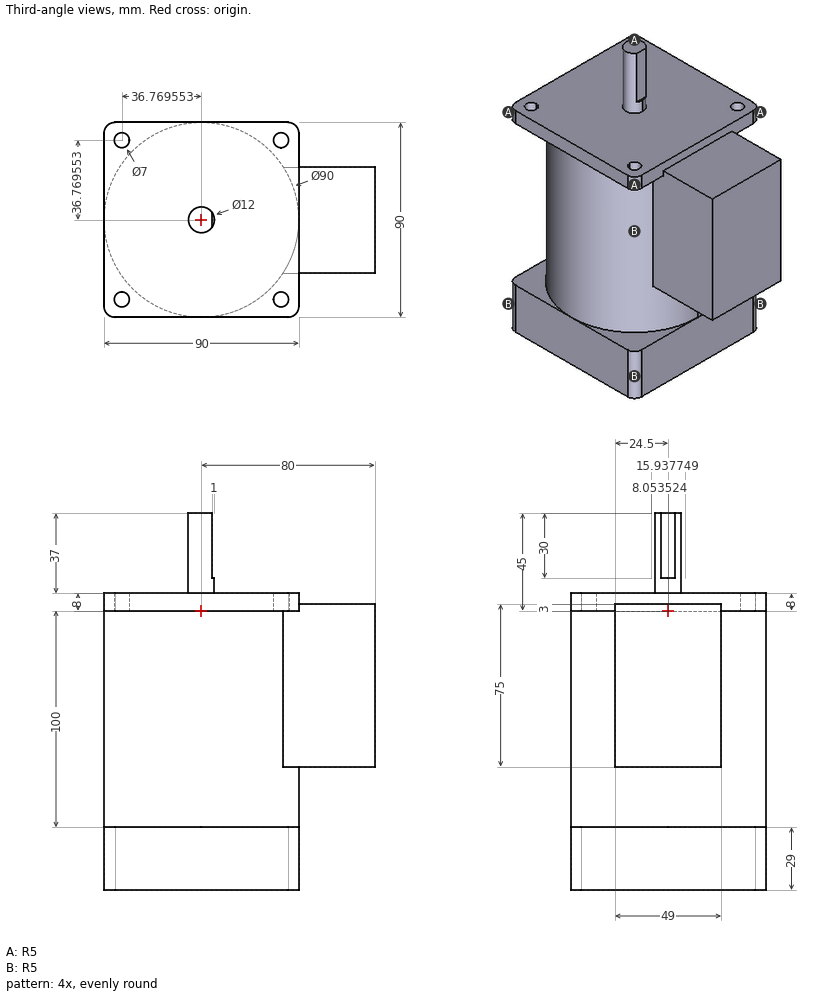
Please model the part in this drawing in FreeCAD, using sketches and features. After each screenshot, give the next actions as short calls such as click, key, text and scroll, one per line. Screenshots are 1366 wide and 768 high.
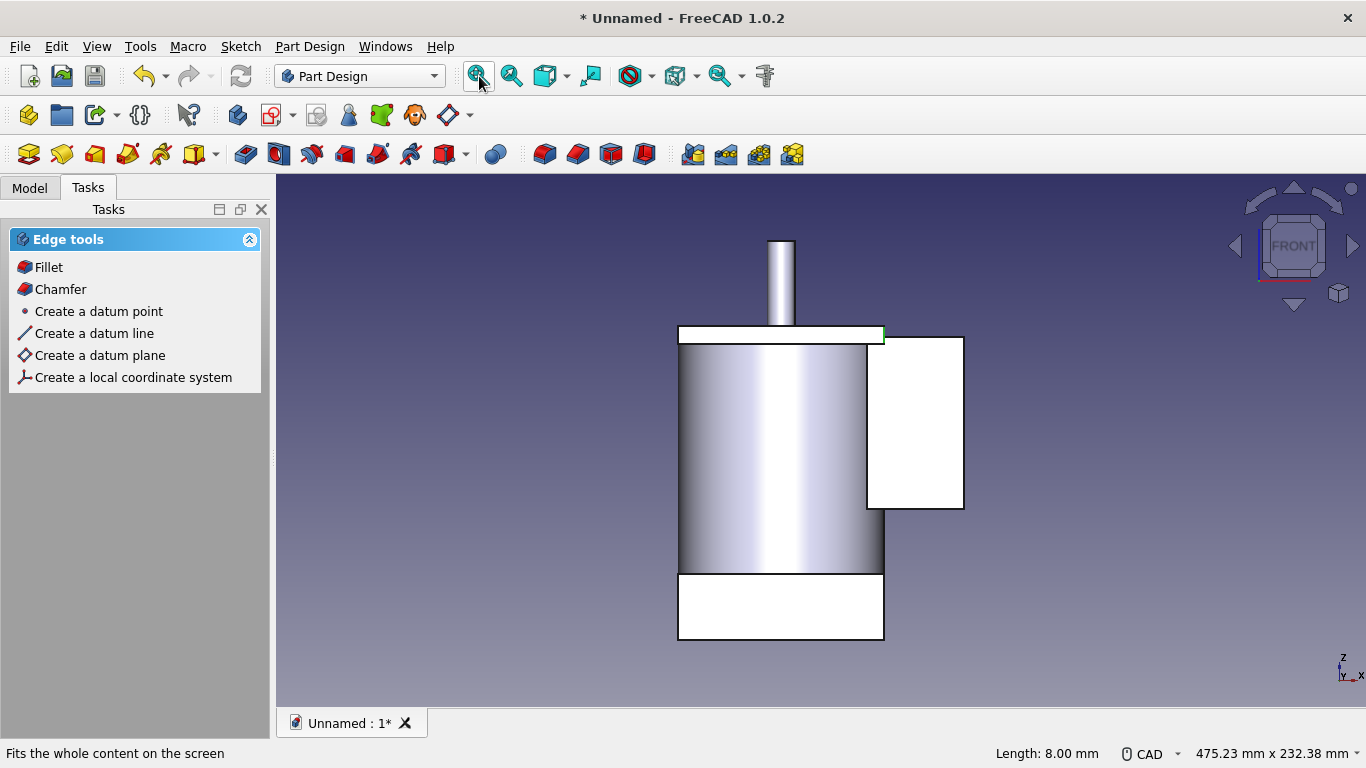
click(678, 334, ctrl)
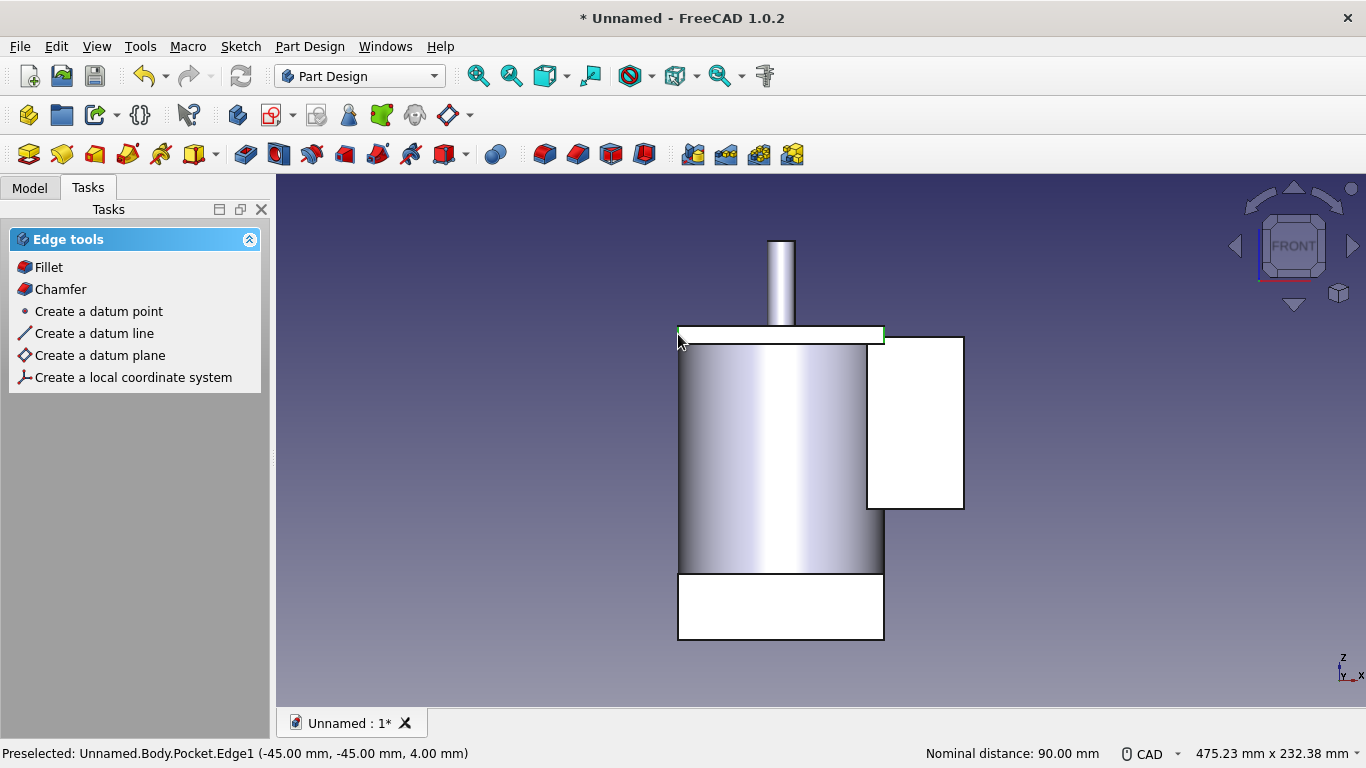
scroll(678, 334, up, 4)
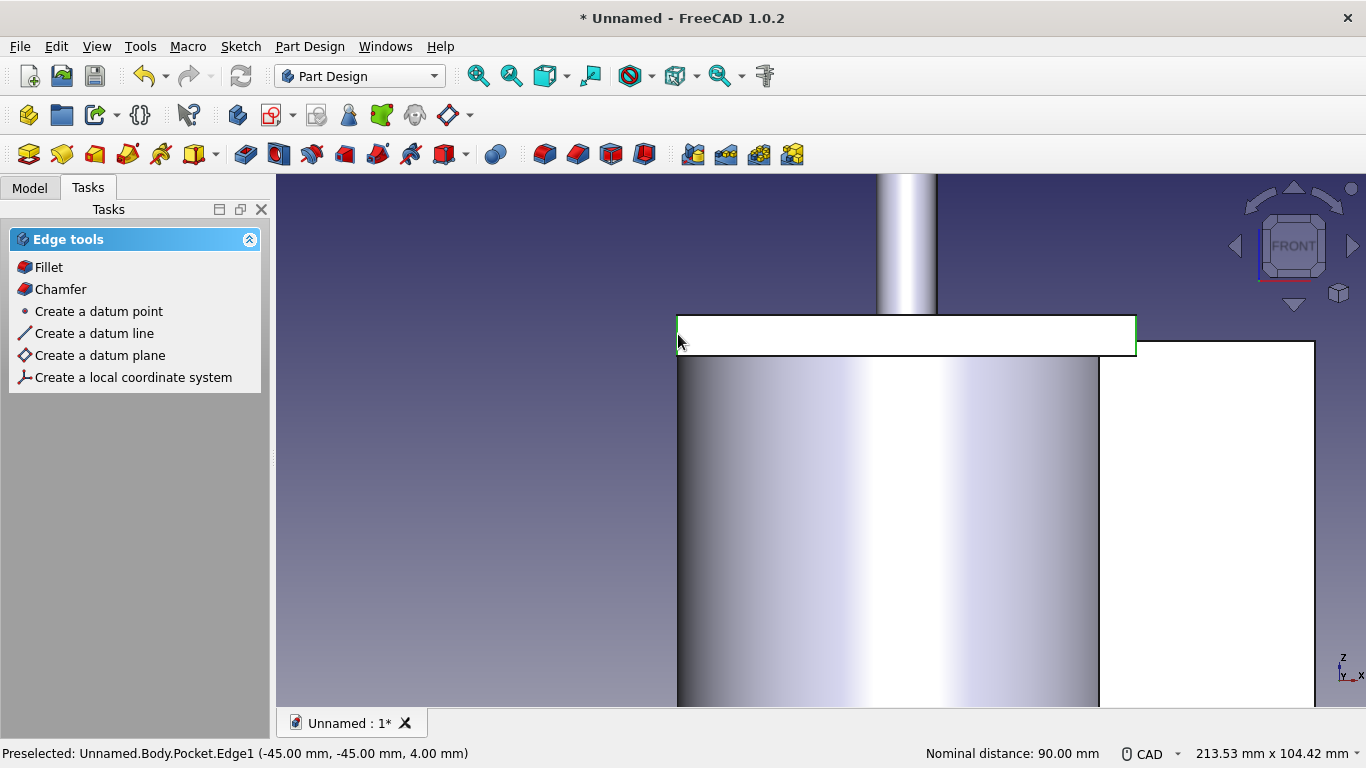
key(v)
key(f)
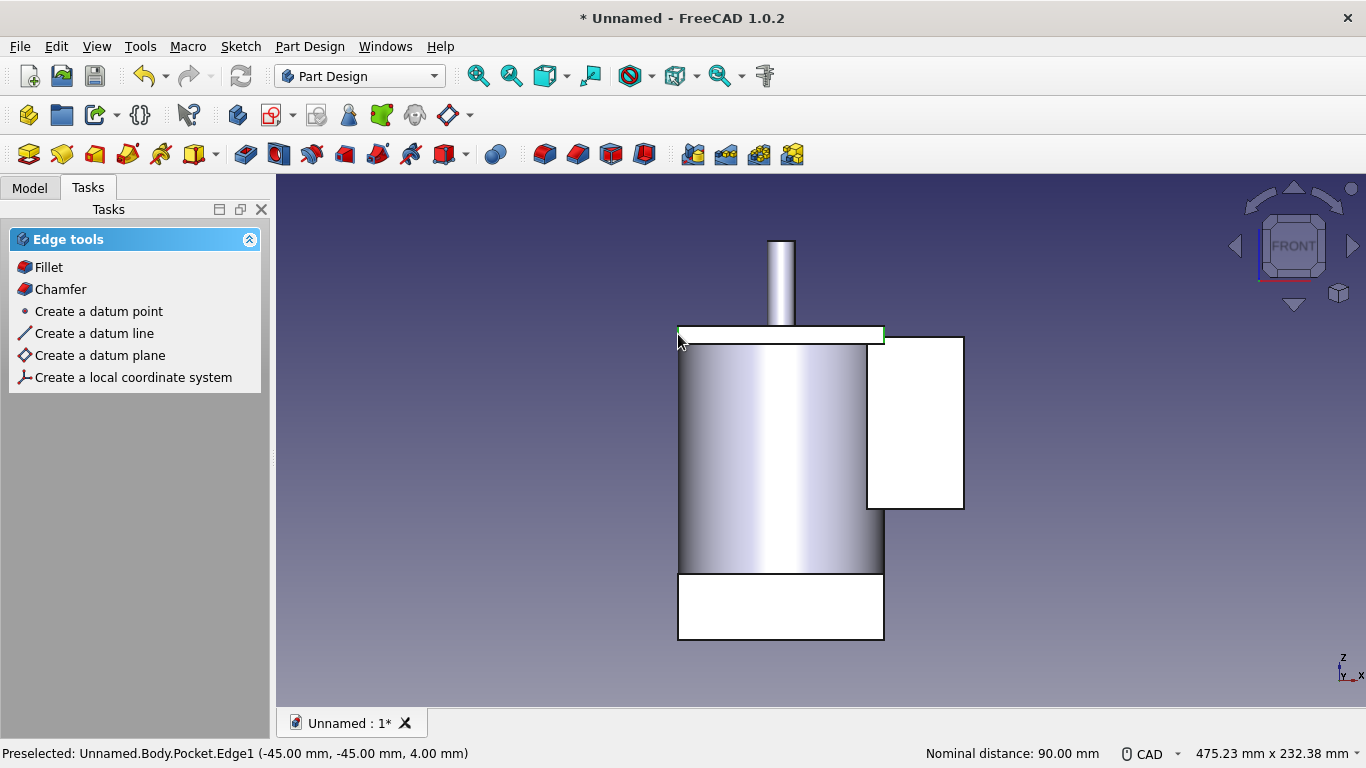
key(3)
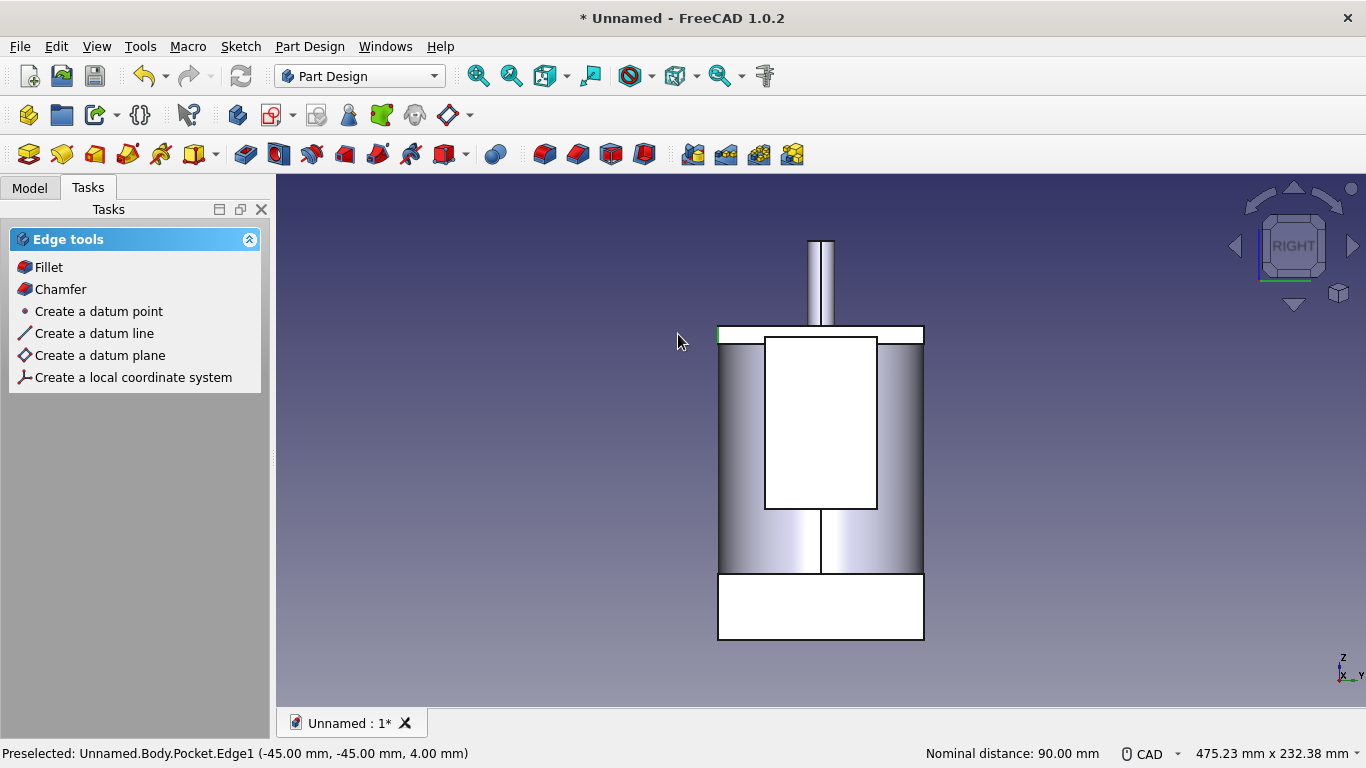
click(924, 334, ctrl)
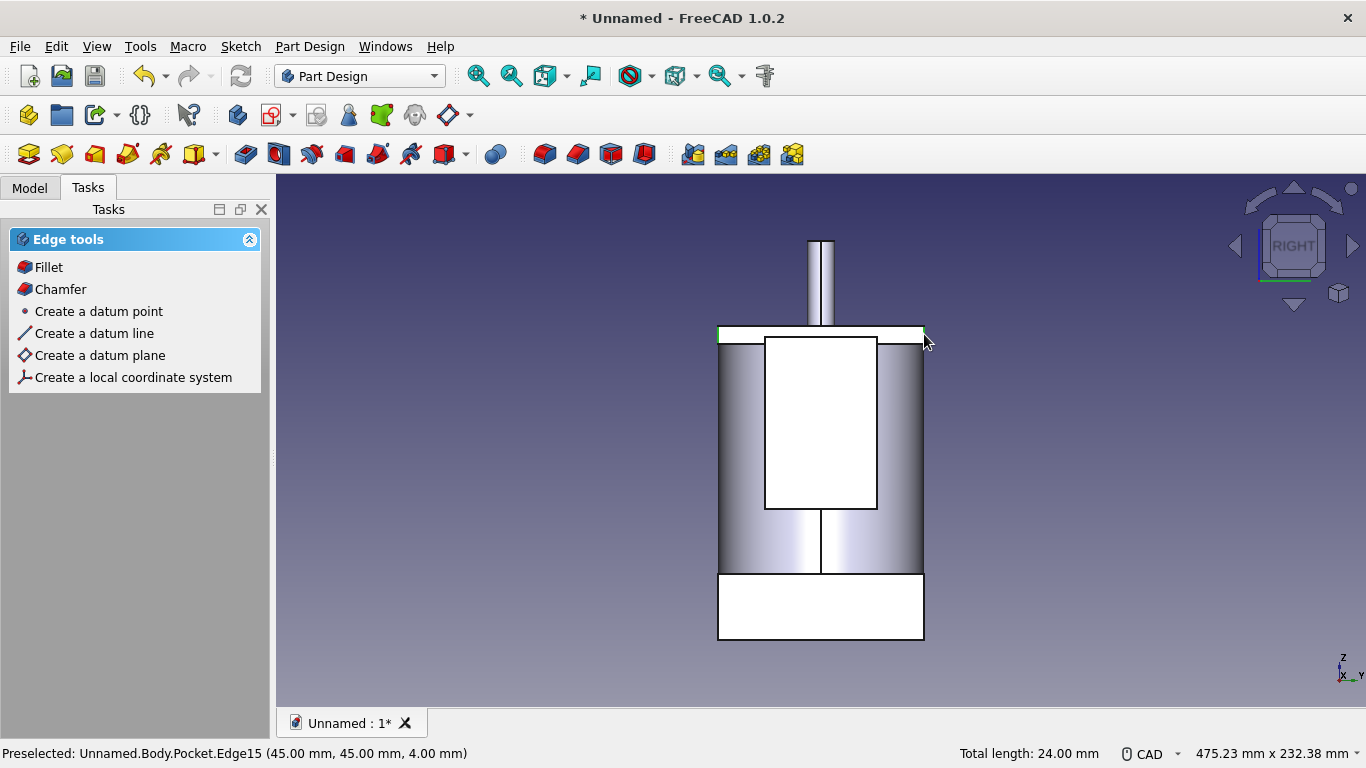
scroll(924, 334, up, 4)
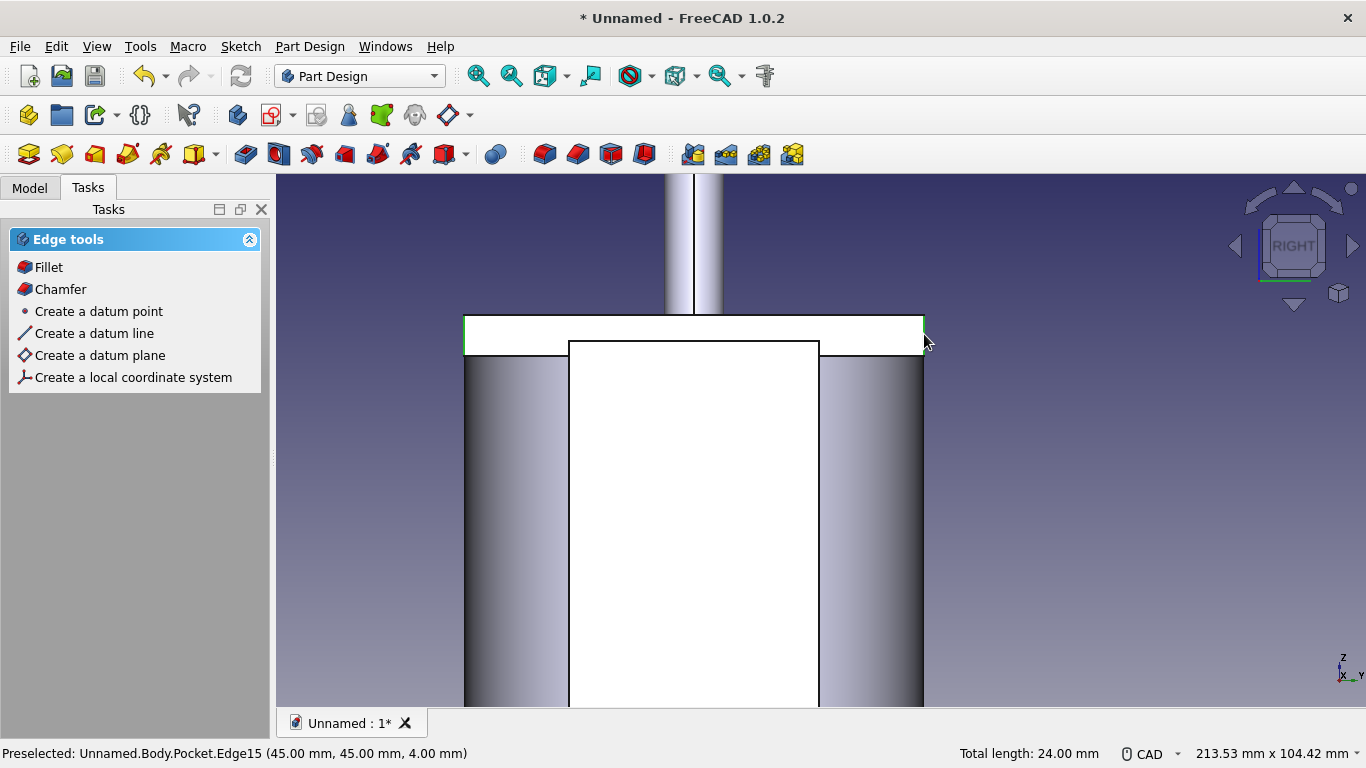
key(v)
key(f)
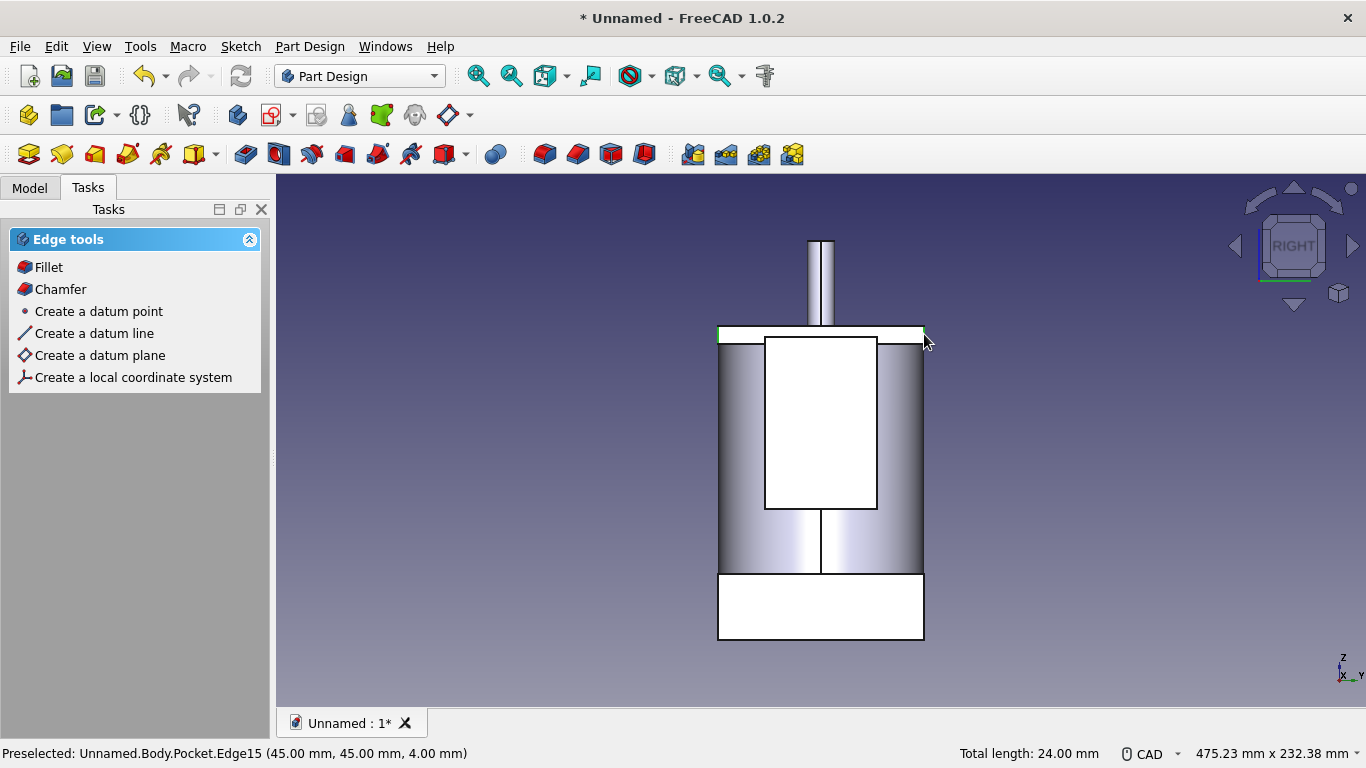
key(5)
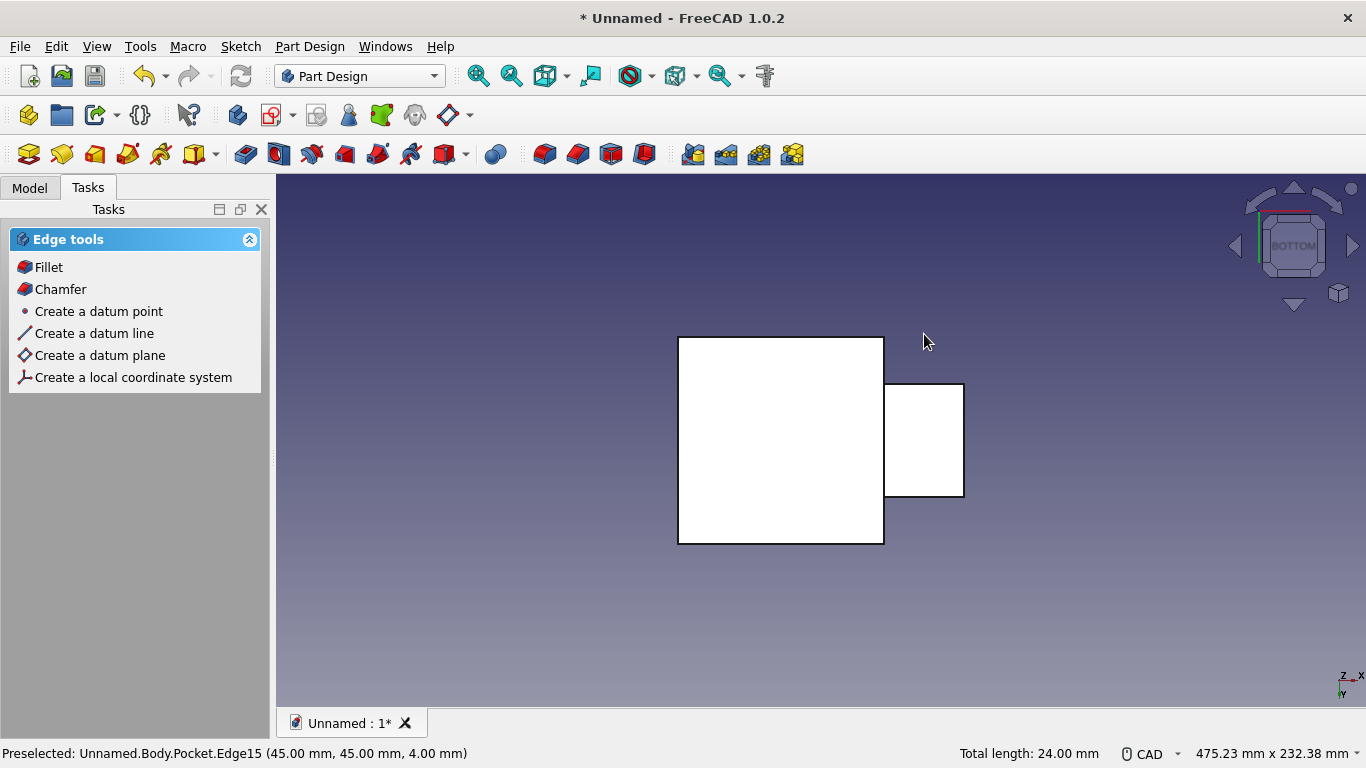
click(479, 76)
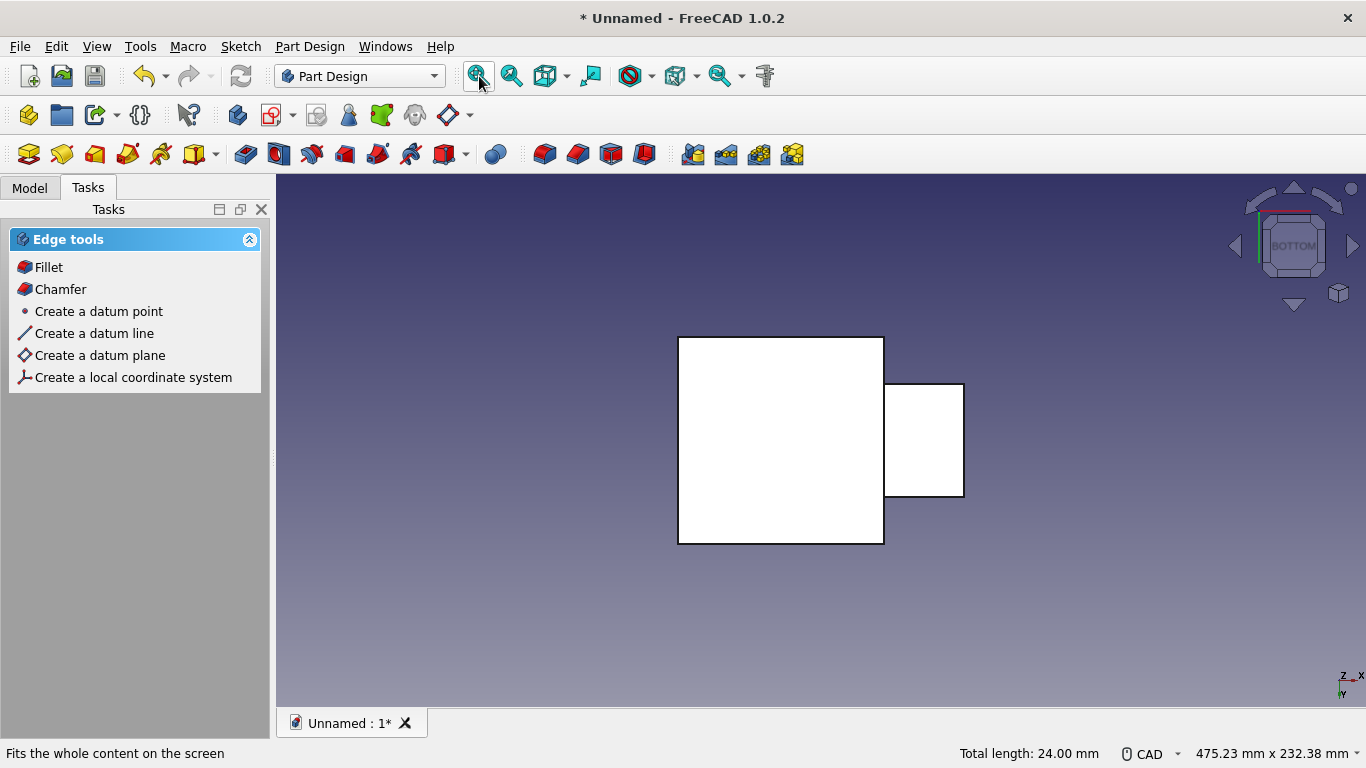
scroll(678, 543, up, 4)